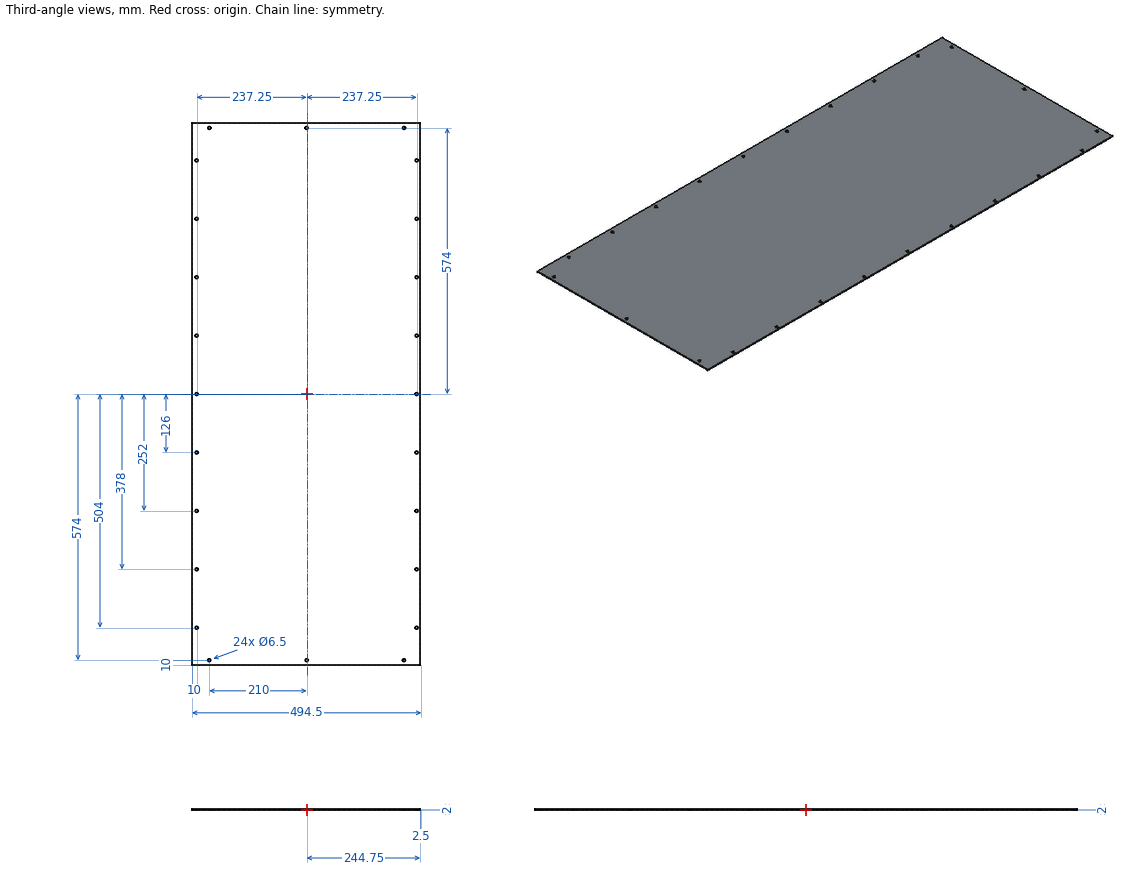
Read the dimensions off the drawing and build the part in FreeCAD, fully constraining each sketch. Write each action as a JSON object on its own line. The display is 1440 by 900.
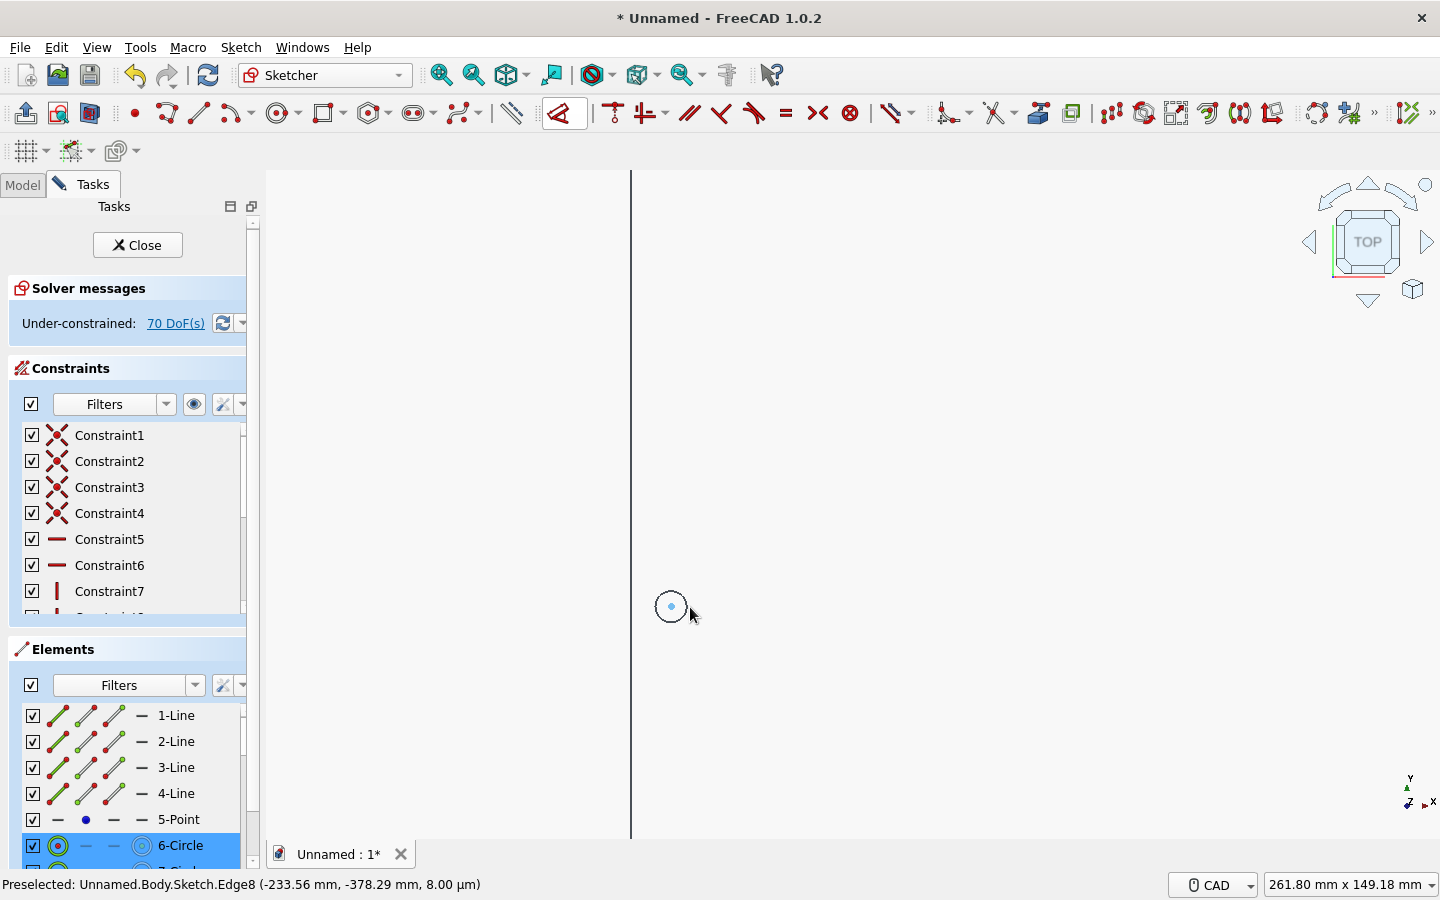
{"action": "left_click", "coordinate": [682, 596]}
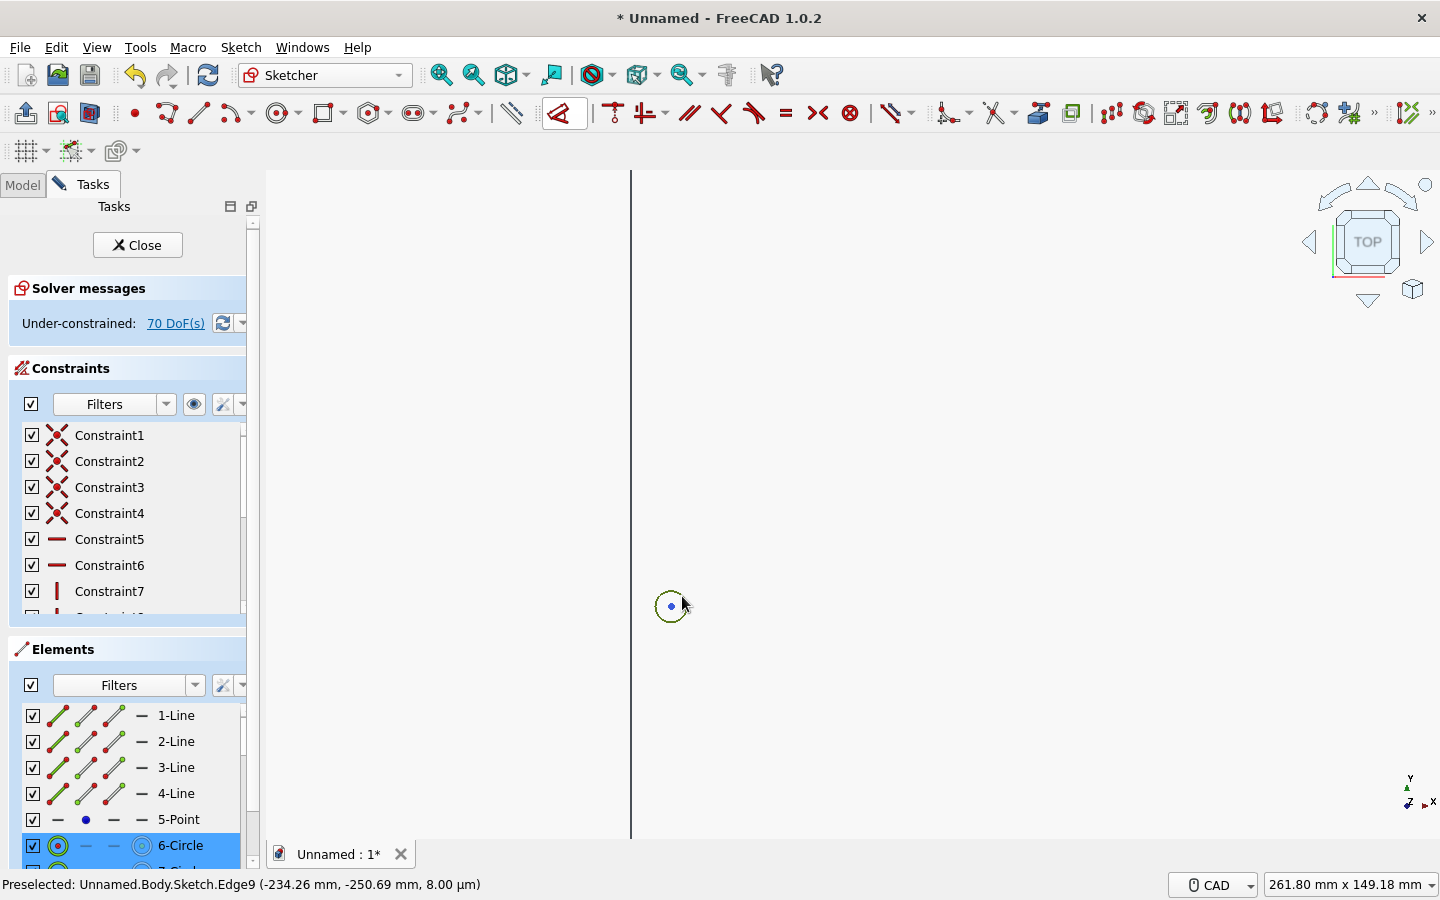
{"action": "scroll", "coordinate": [690, 607], "scroll_direction": "down", "scroll_amount": 12}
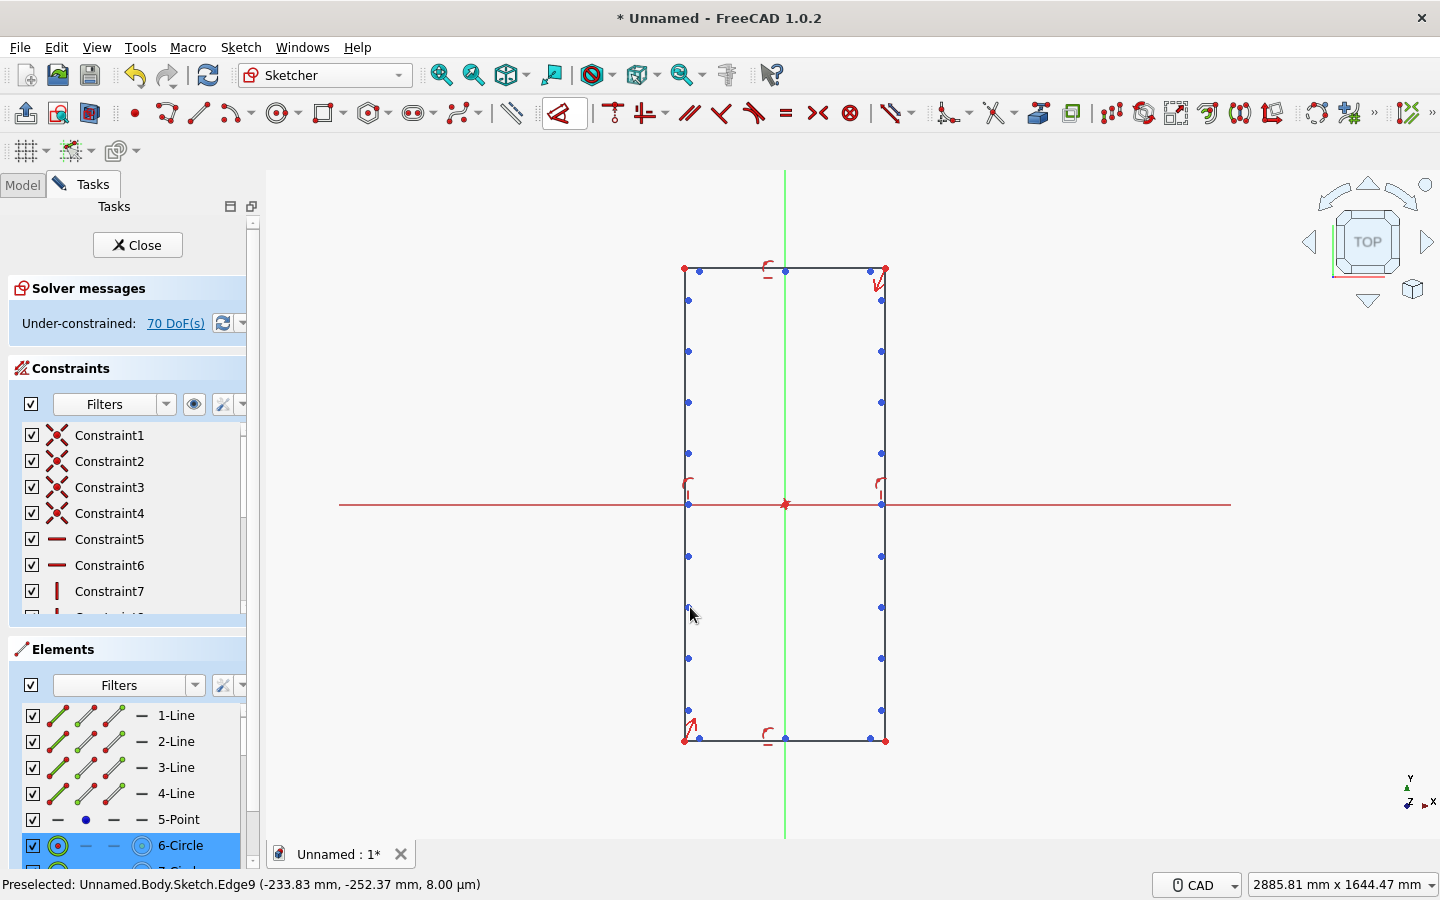
{"action": "scroll", "coordinate": [690, 555], "scroll_direction": "up", "scroll_amount": 11}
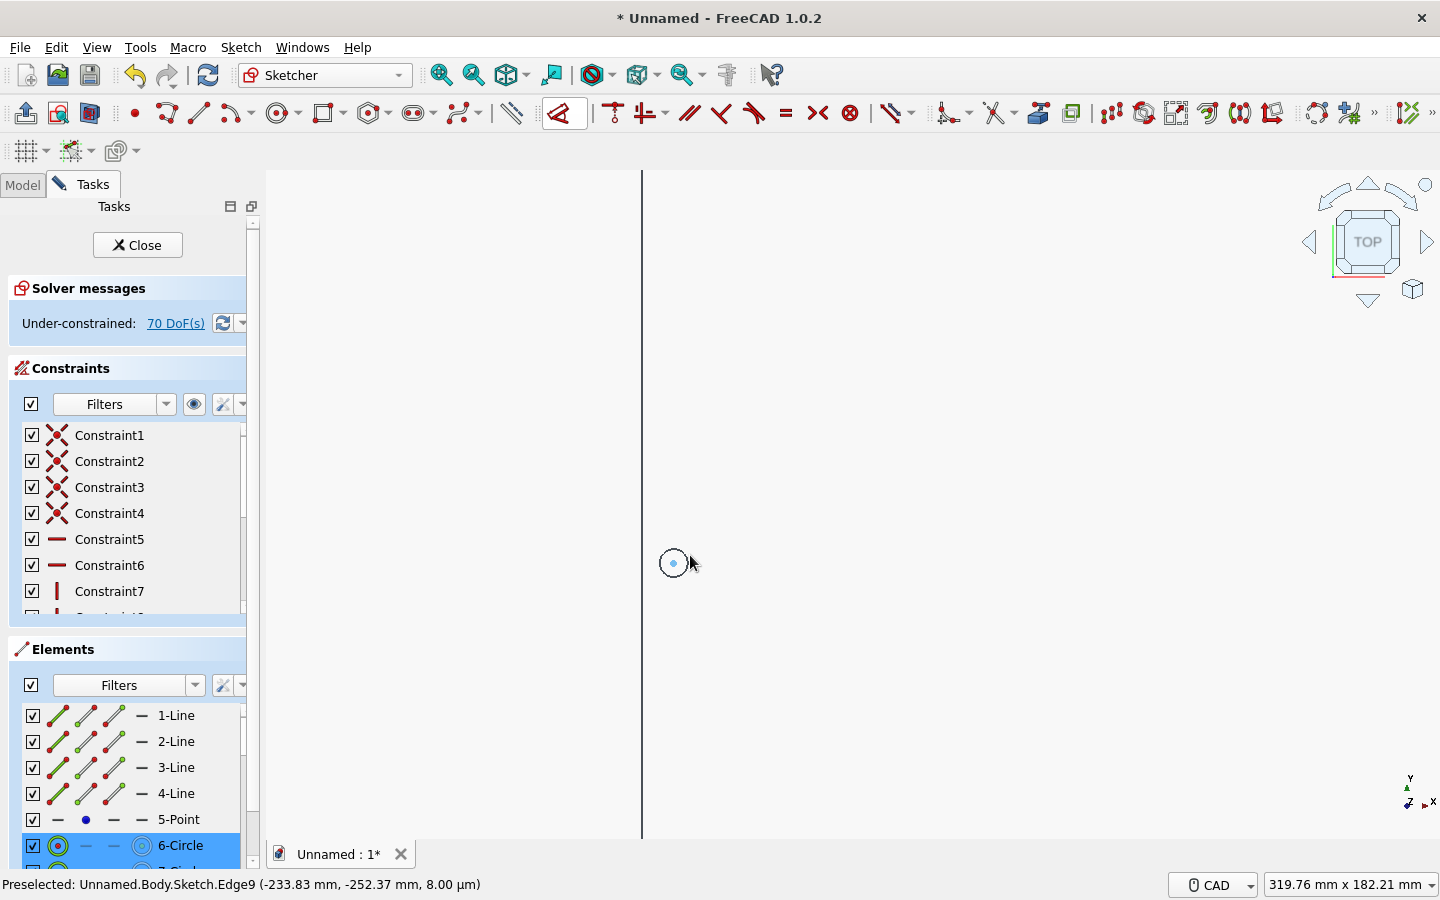
{"action": "left_click", "coordinate": [684, 553]}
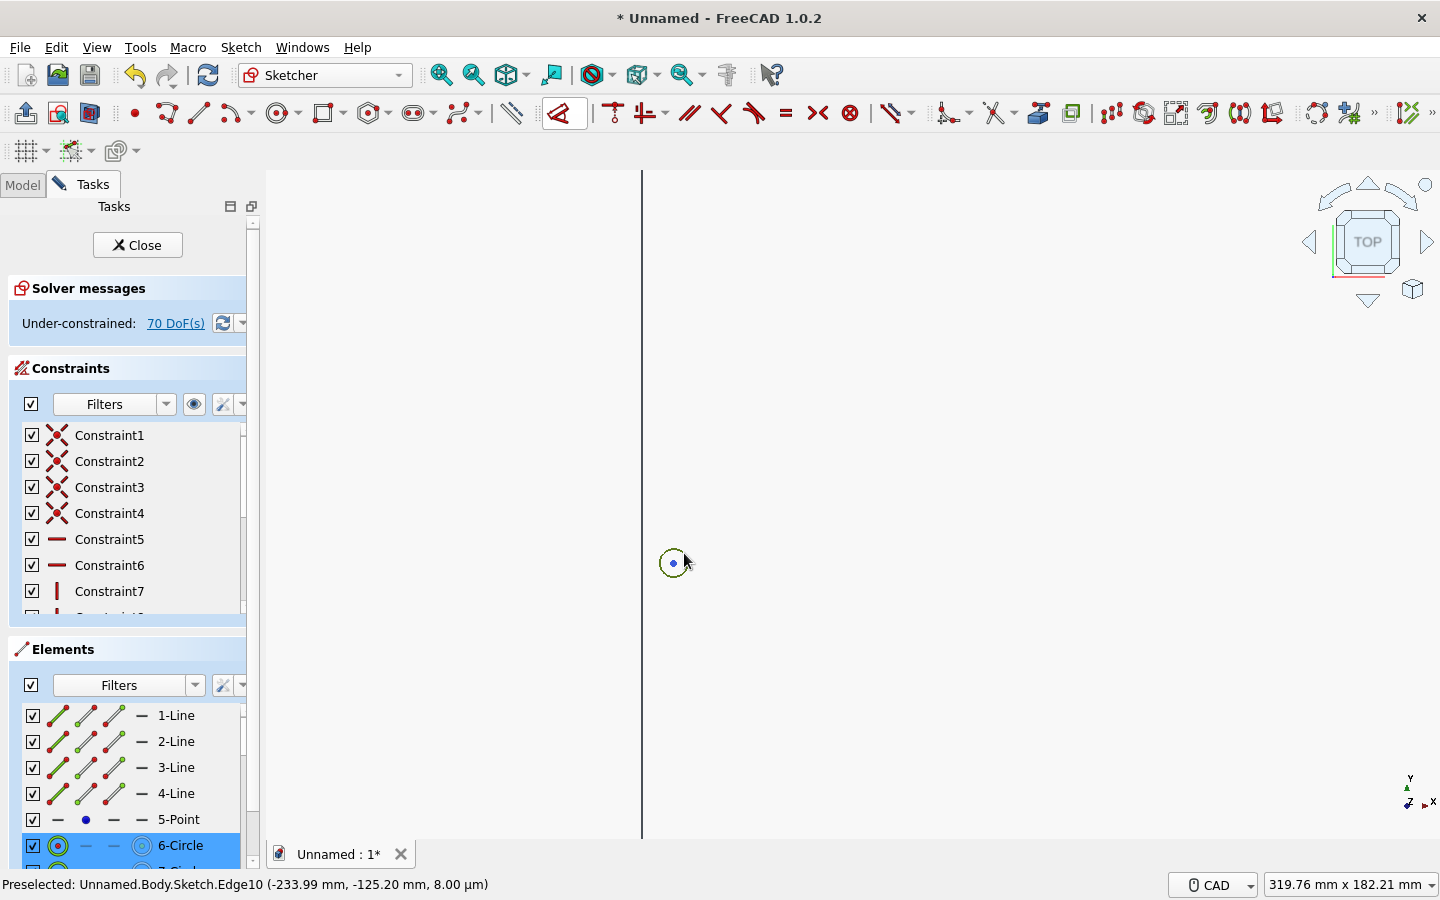
{"action": "scroll", "coordinate": [690, 555], "scroll_direction": "down", "scroll_amount": 11}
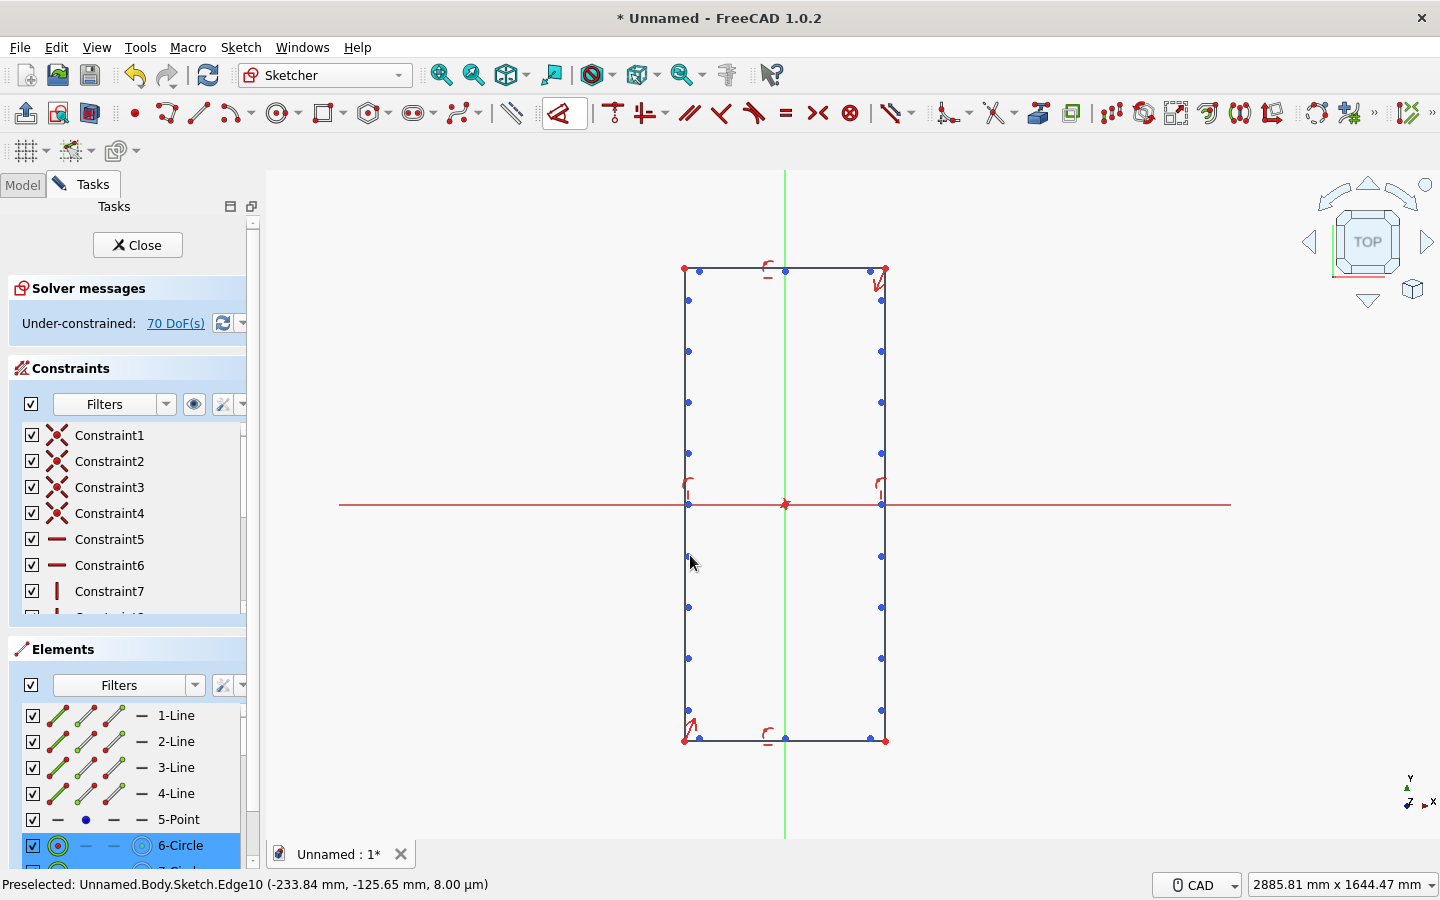
{"action": "scroll", "coordinate": [785, 737], "scroll_direction": "up", "scroll_amount": 12}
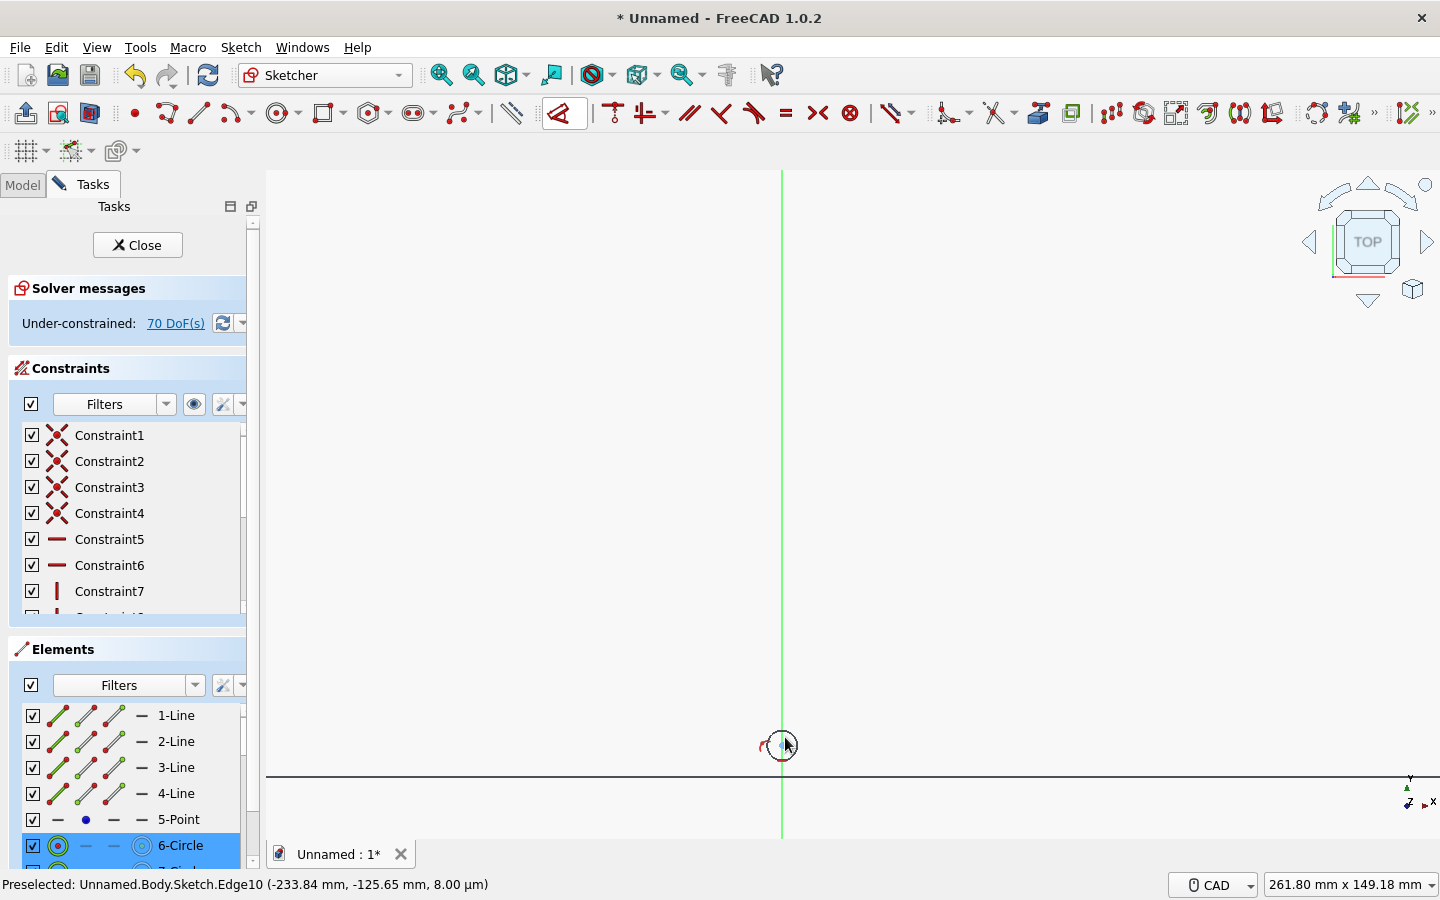
{"action": "left_click", "coordinate": [783, 731]}